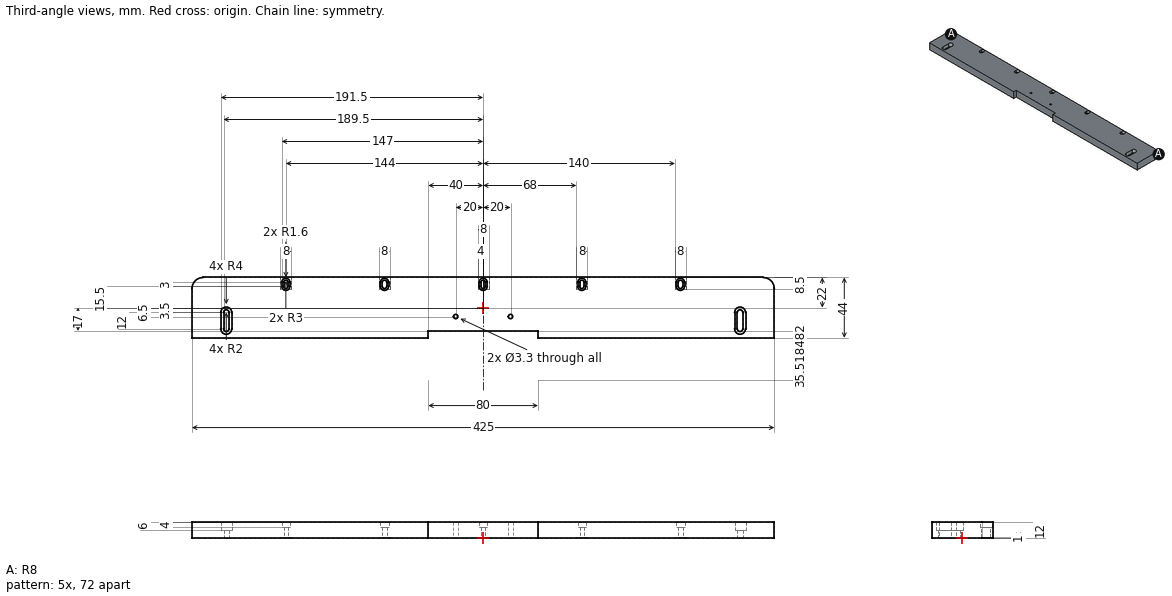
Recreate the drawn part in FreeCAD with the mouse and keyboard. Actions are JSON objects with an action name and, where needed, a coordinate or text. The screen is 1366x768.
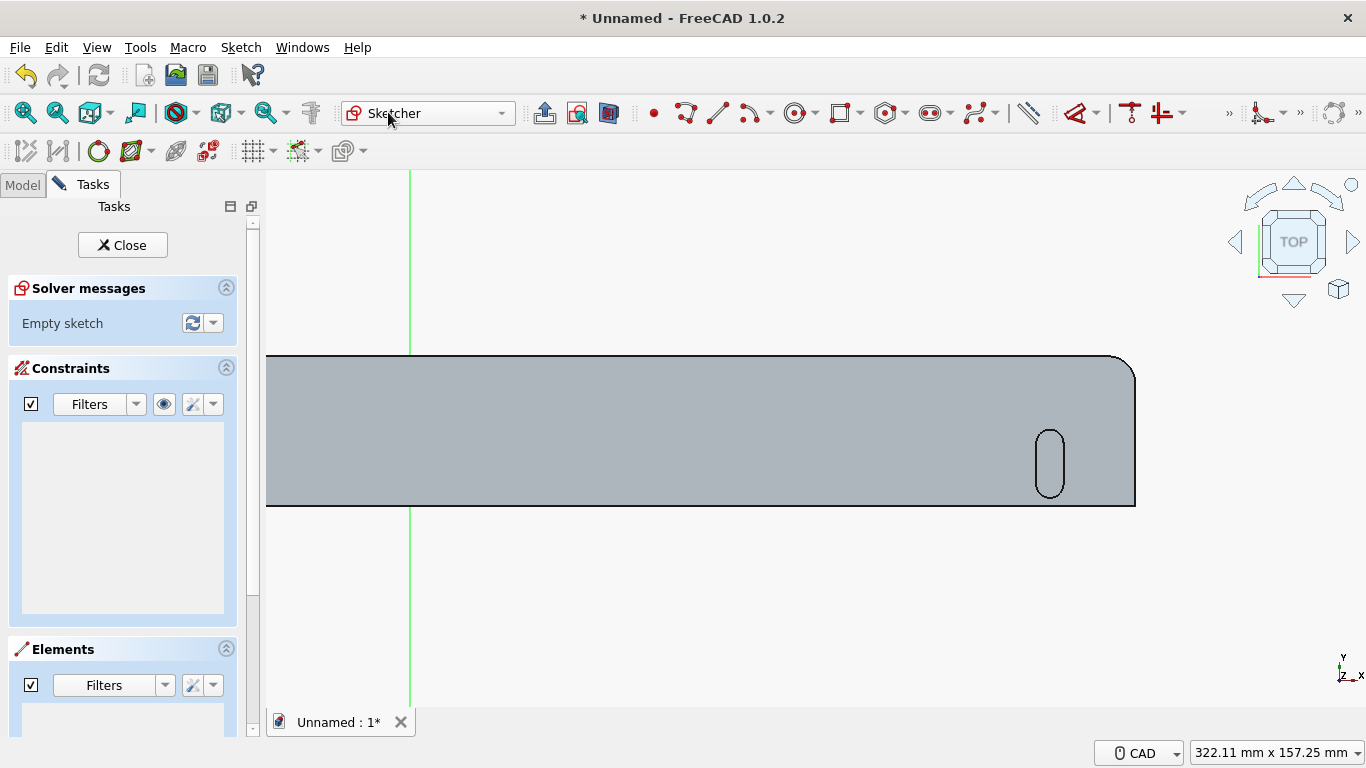
{"action": "scroll", "coordinate": [1023, 420], "scroll_direction": "down", "scroll_amount": 4}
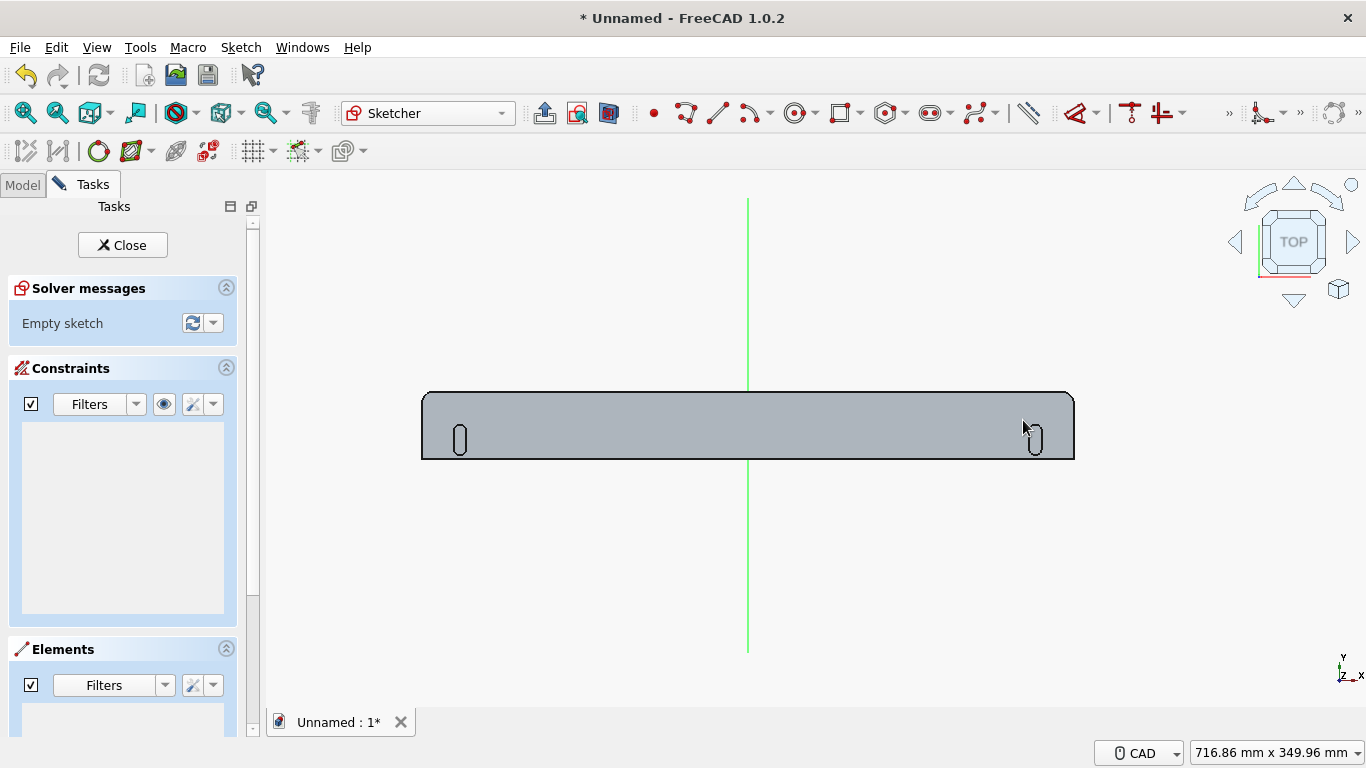
{"action": "left_click", "coordinate": [930, 114]}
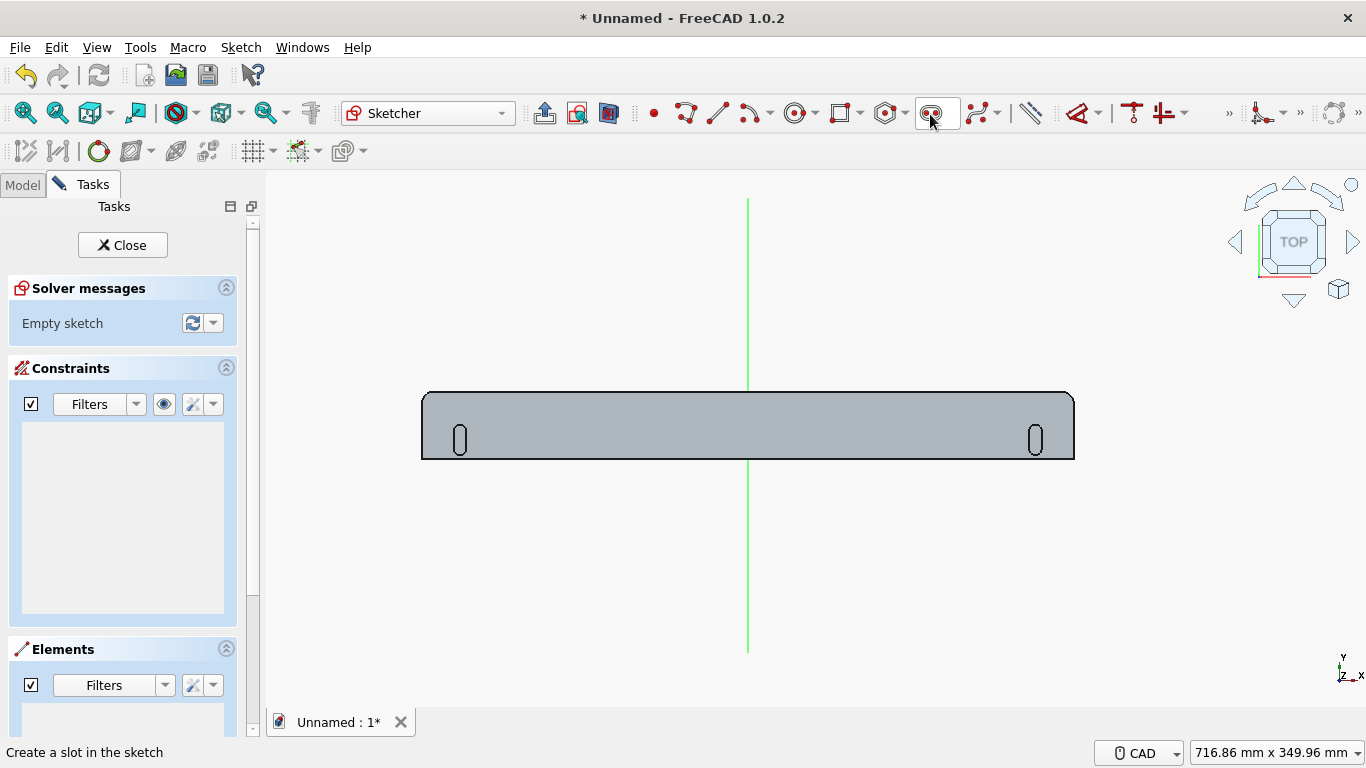
{"action": "scroll", "coordinate": [460, 449], "scroll_direction": "up", "scroll_amount": 11}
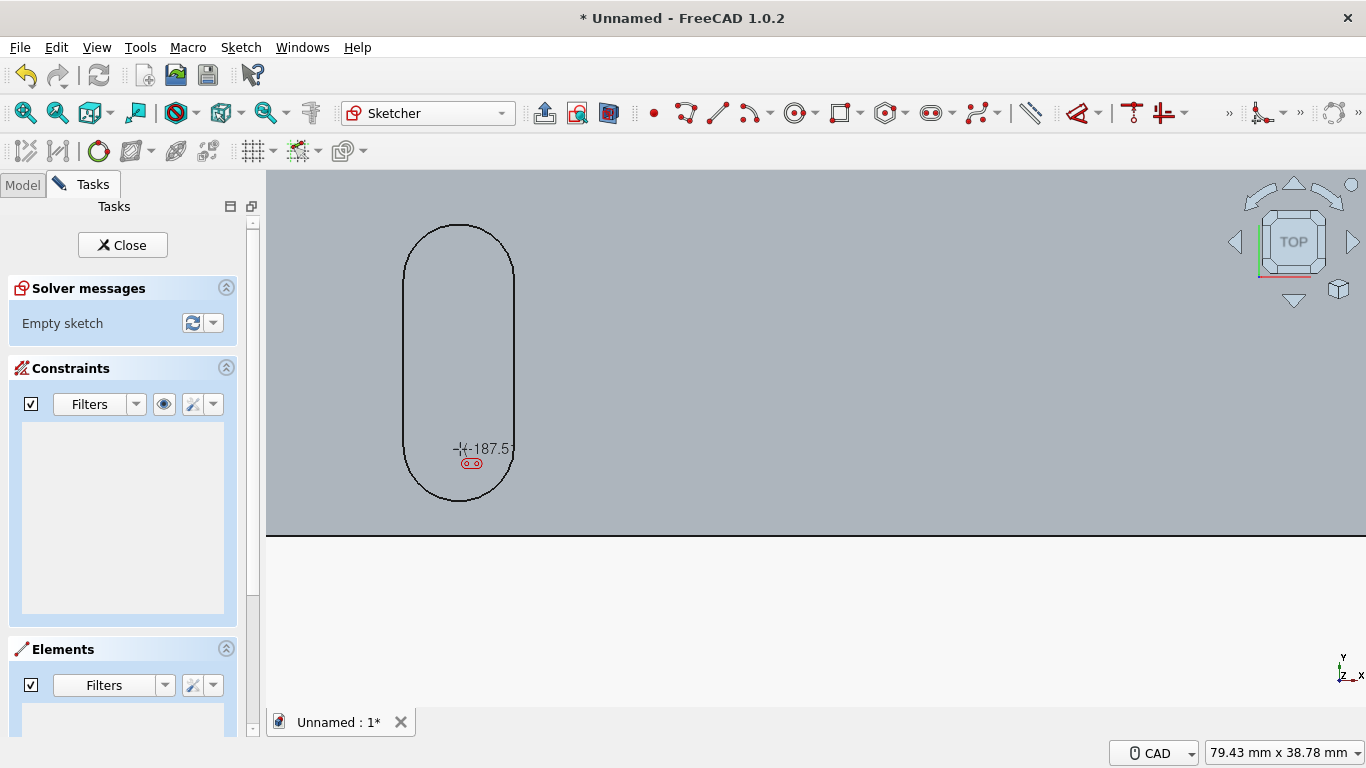
{"action": "scroll", "coordinate": [460, 449], "scroll_direction": "down", "scroll_amount": 11}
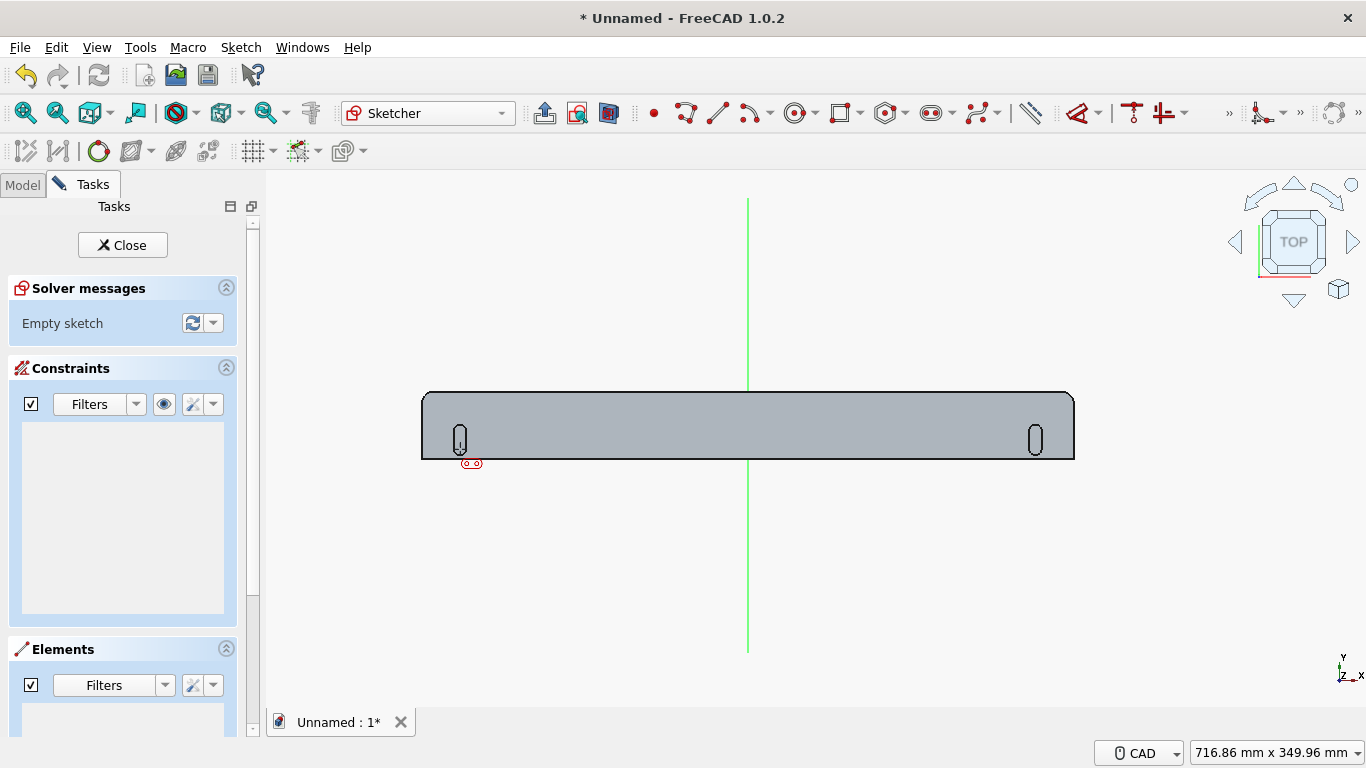
{"action": "left_click", "coordinate": [460, 449]}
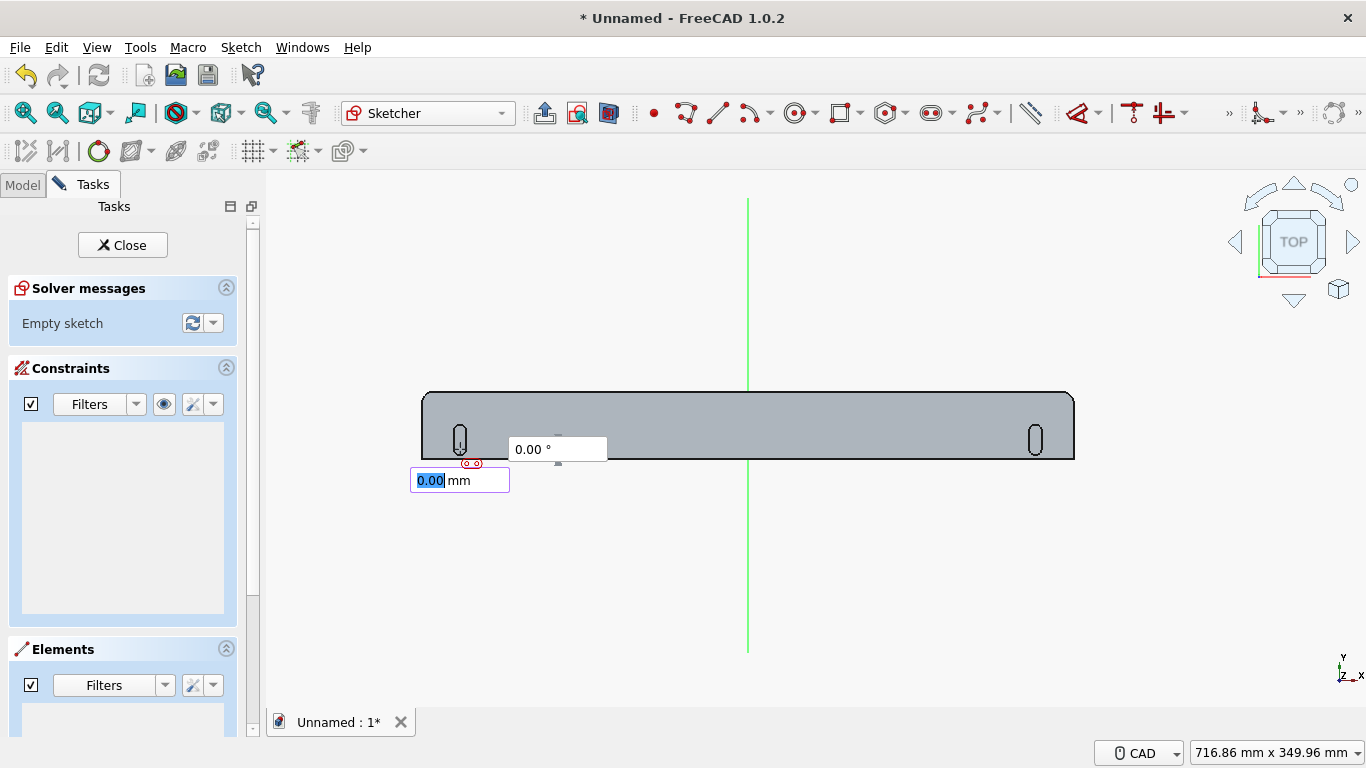
{"action": "scroll", "coordinate": [460, 431], "scroll_direction": "up", "scroll_amount": 6}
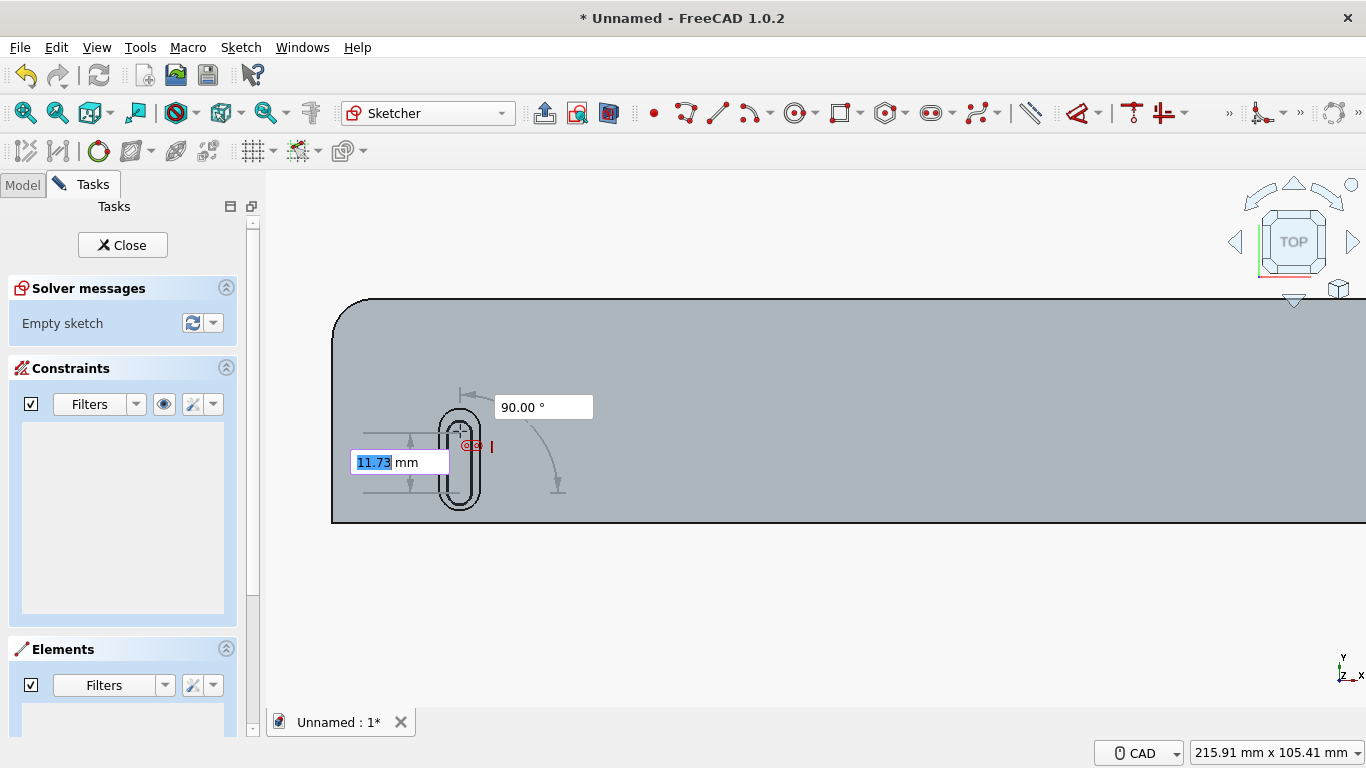
{"action": "left_click", "coordinate": [460, 429]}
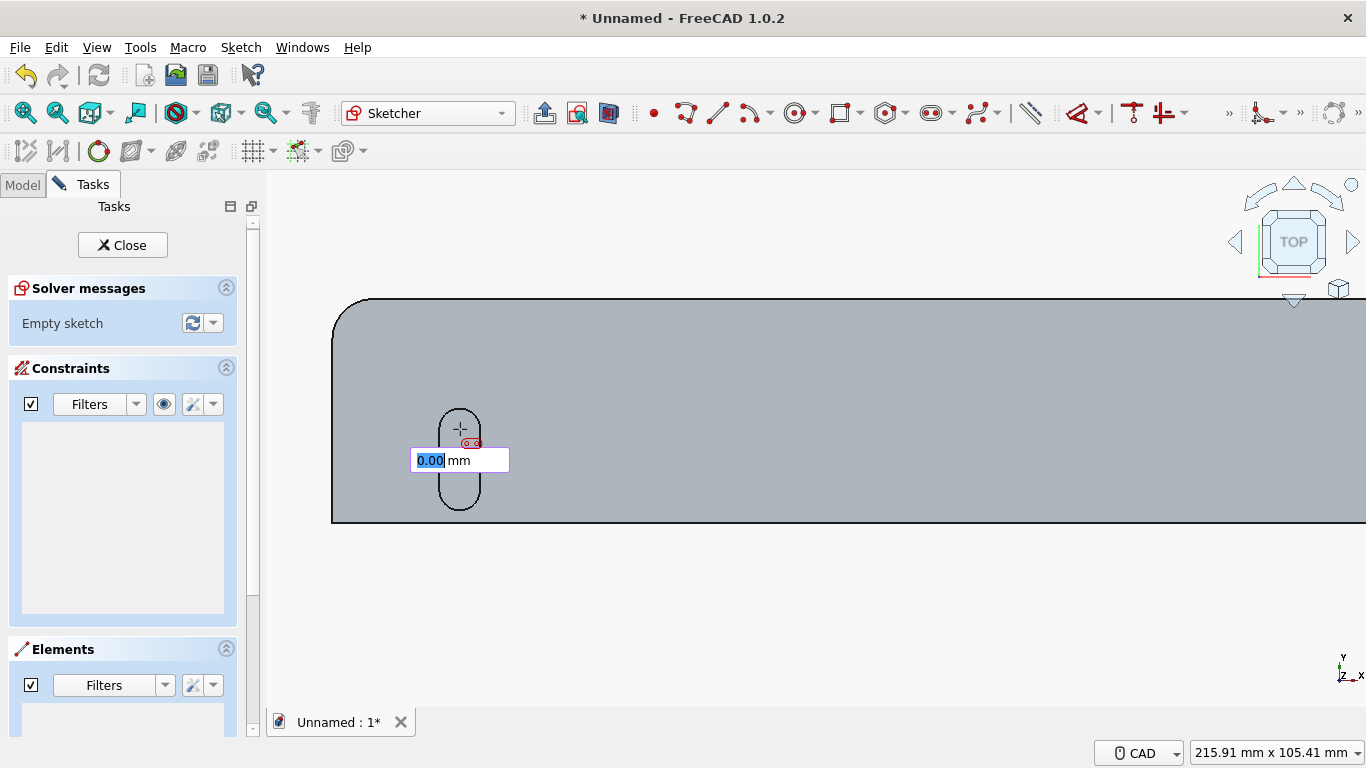
{"action": "scroll", "coordinate": [470, 459], "scroll_direction": "up", "scroll_amount": 3}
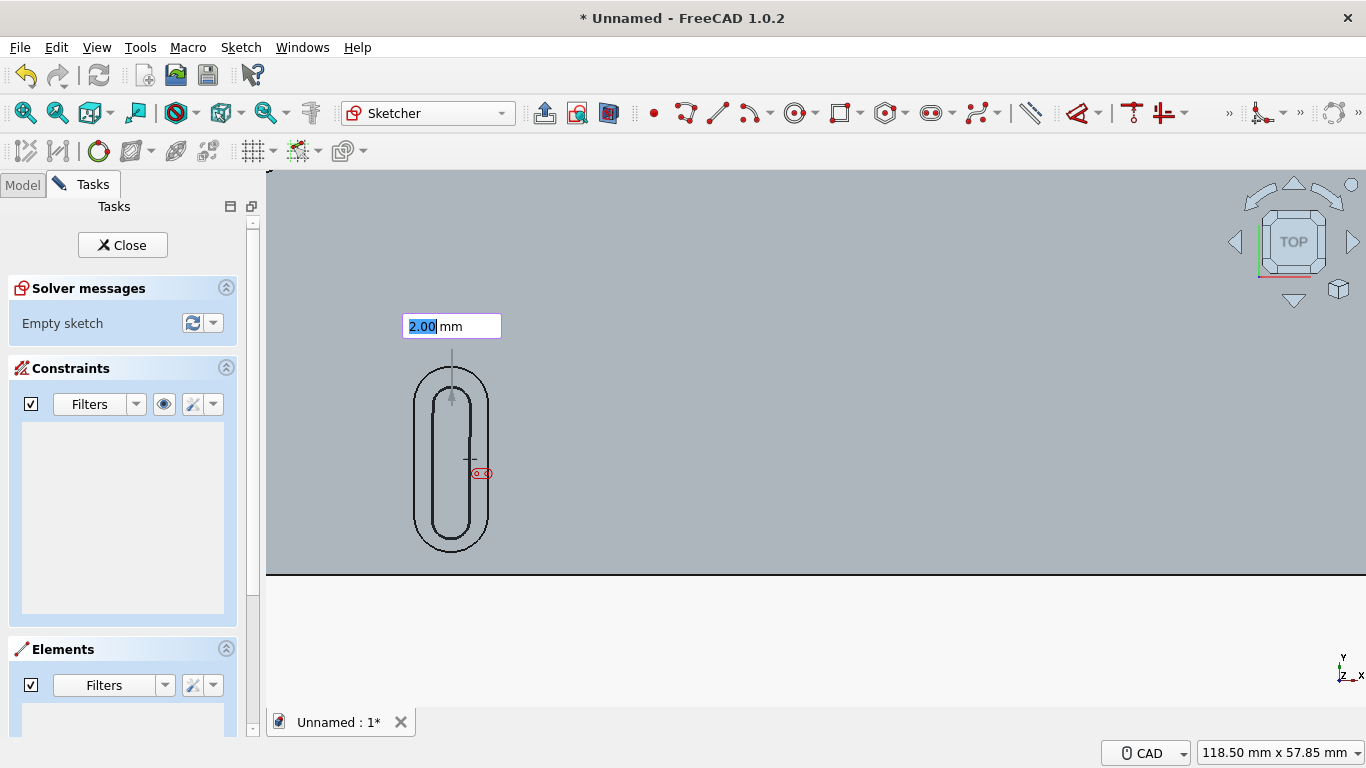
{"action": "left_click", "coordinate": [470, 459]}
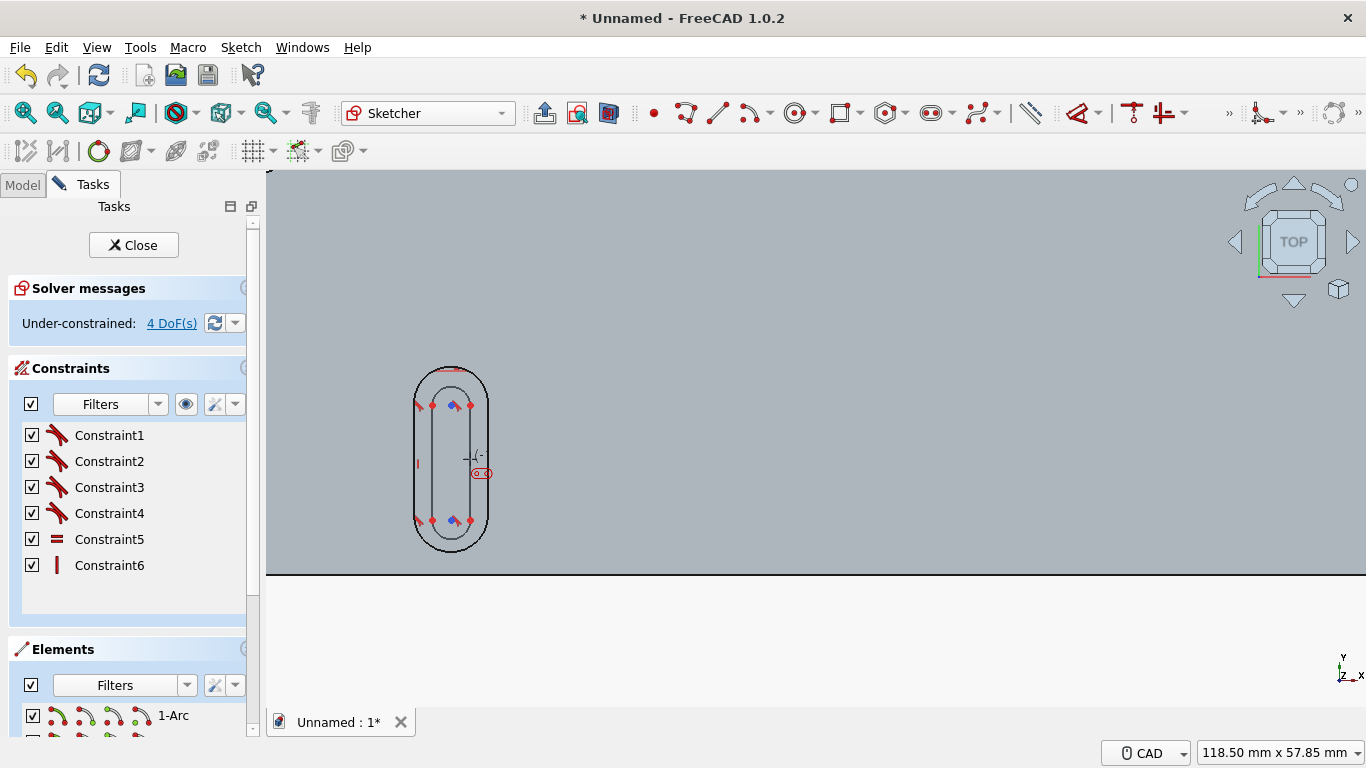
{"action": "scroll", "coordinate": [462, 436], "scroll_direction": "down", "scroll_amount": 9}